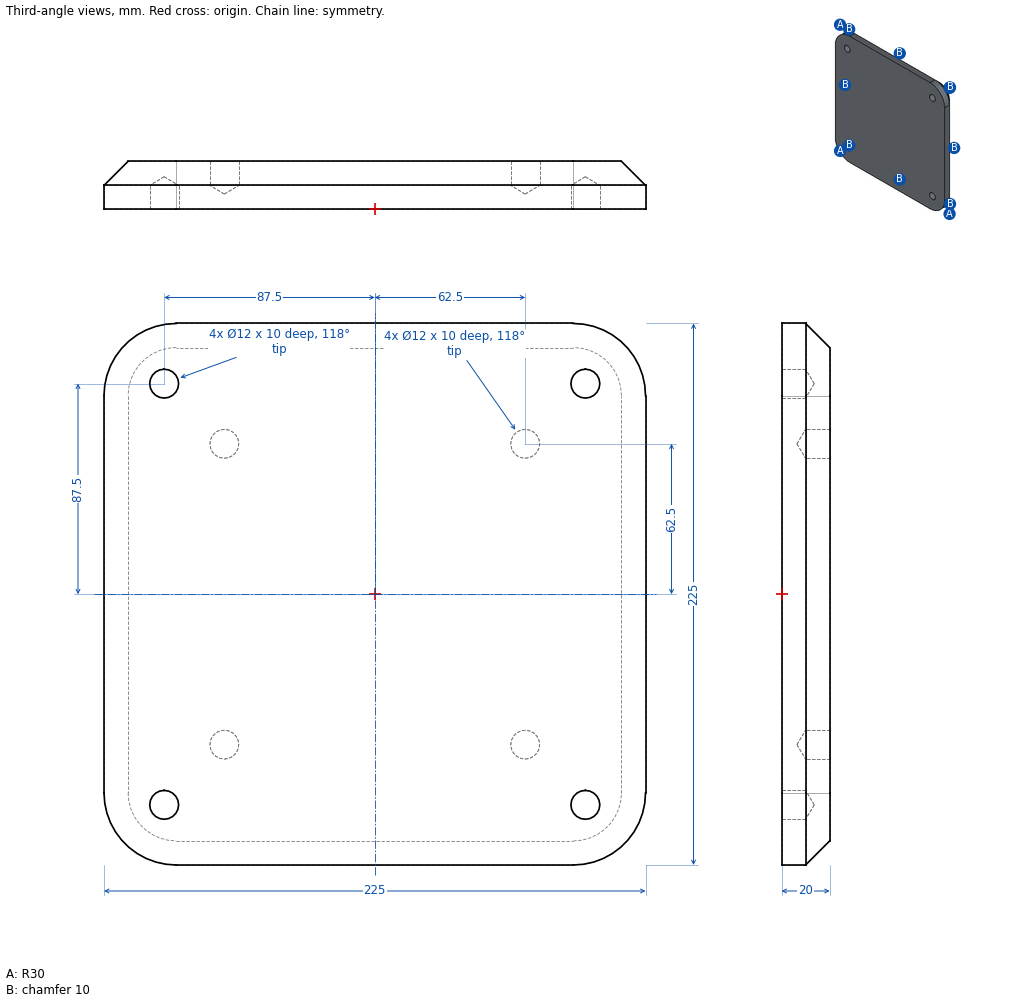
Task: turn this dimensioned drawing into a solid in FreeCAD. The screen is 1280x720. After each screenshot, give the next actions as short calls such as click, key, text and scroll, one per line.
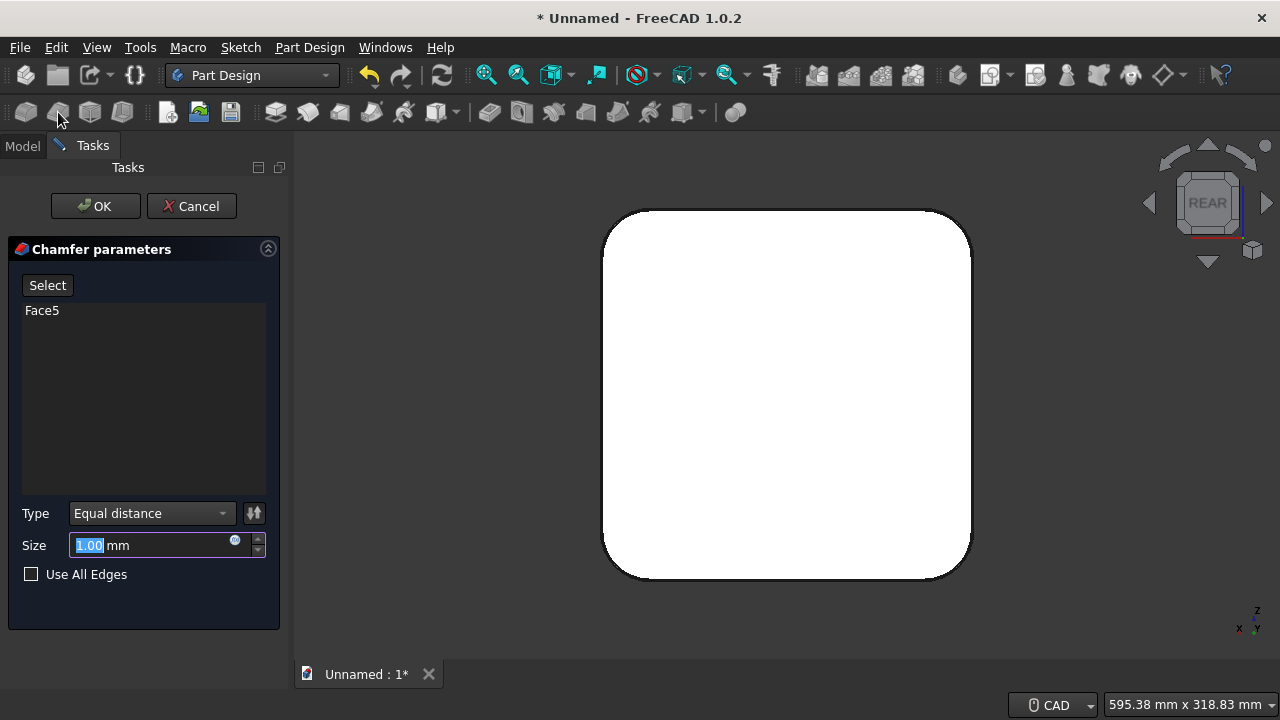
text(10)
key(Tab)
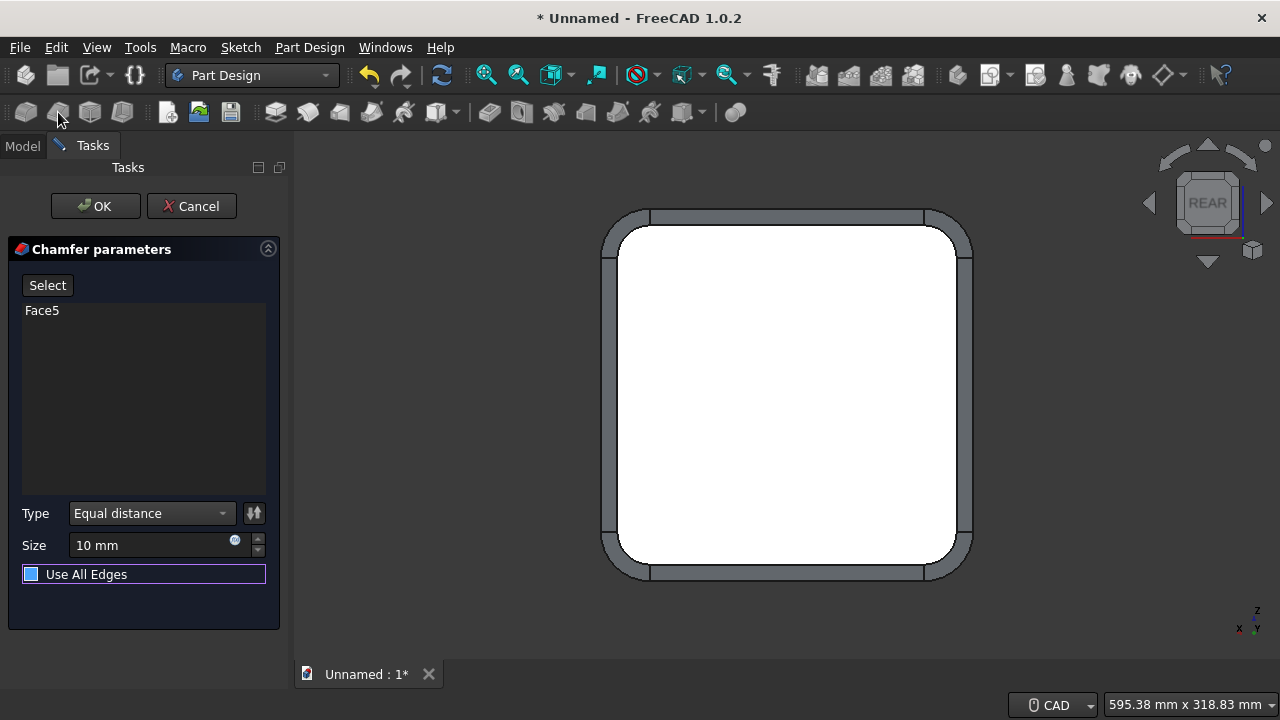
click(96, 206)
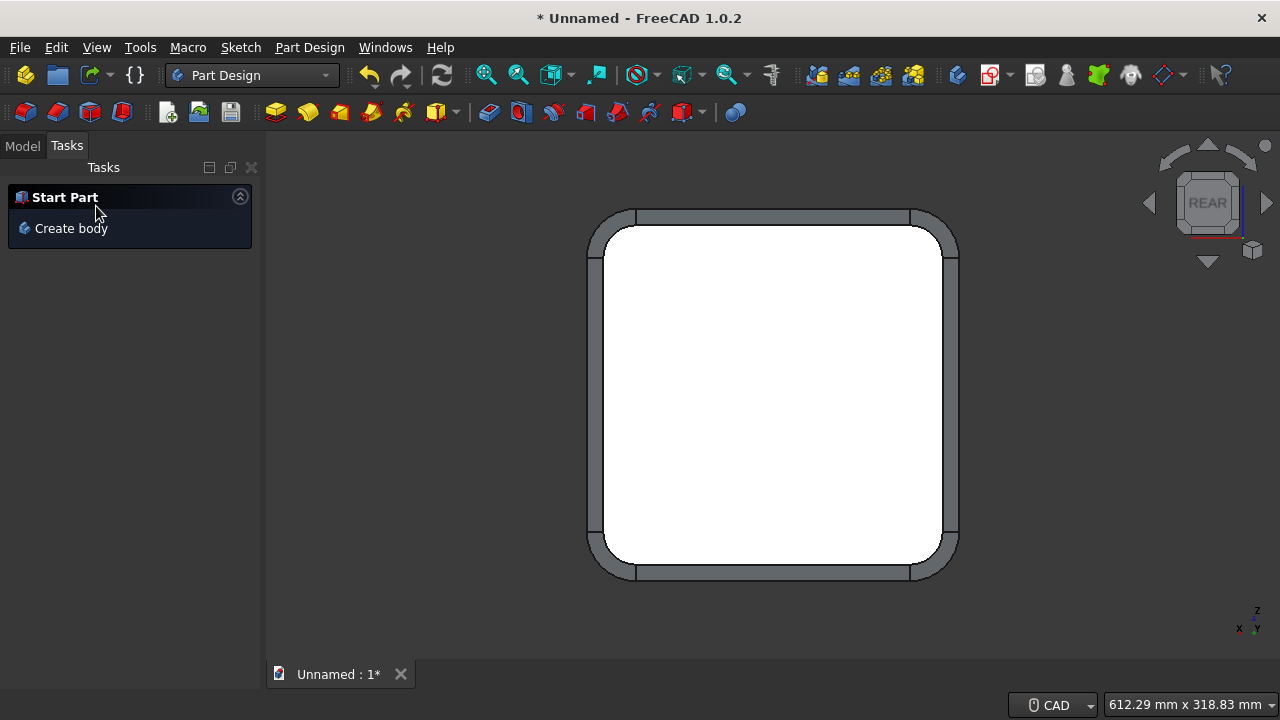
click(773, 394)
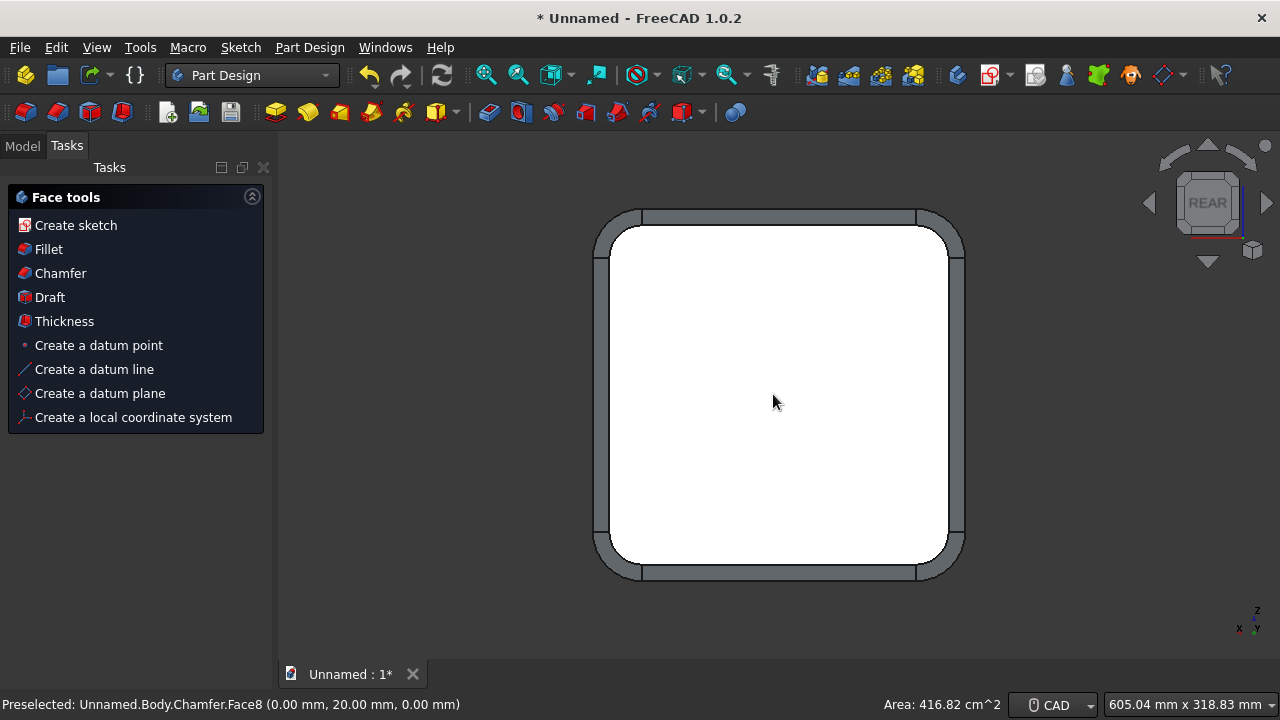
click(990, 76)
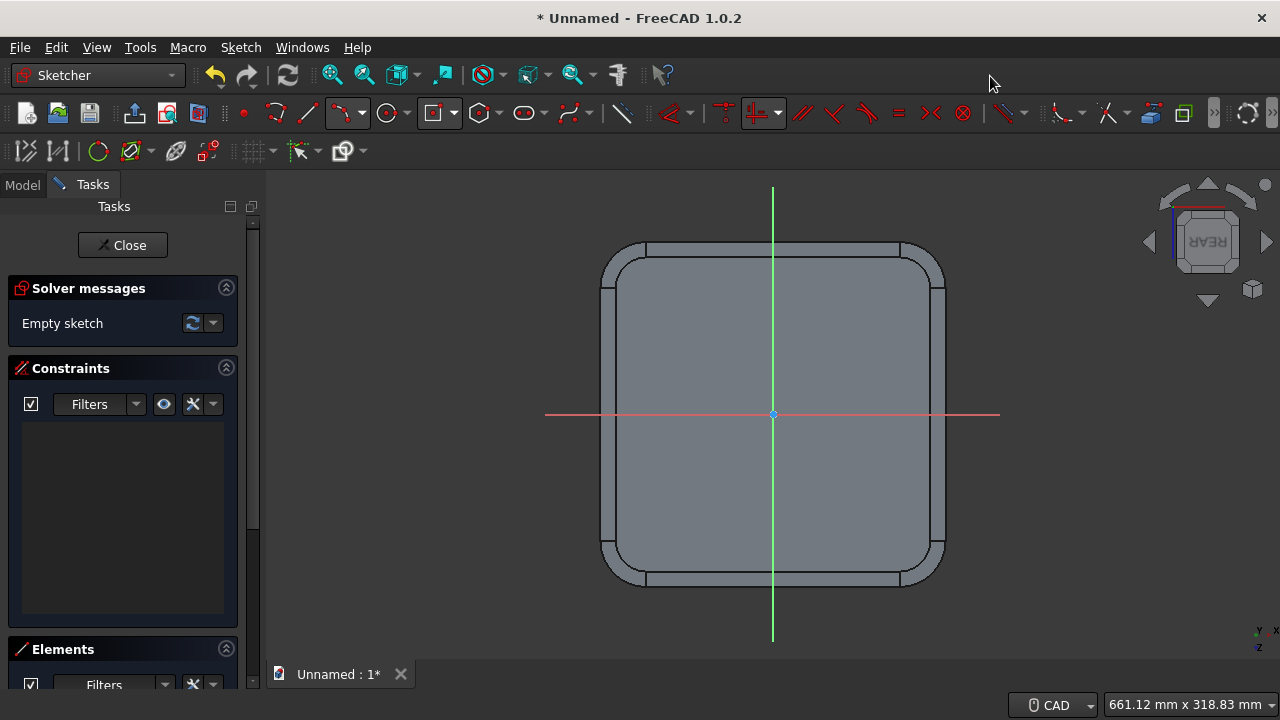
scroll(912, 415, up, 2)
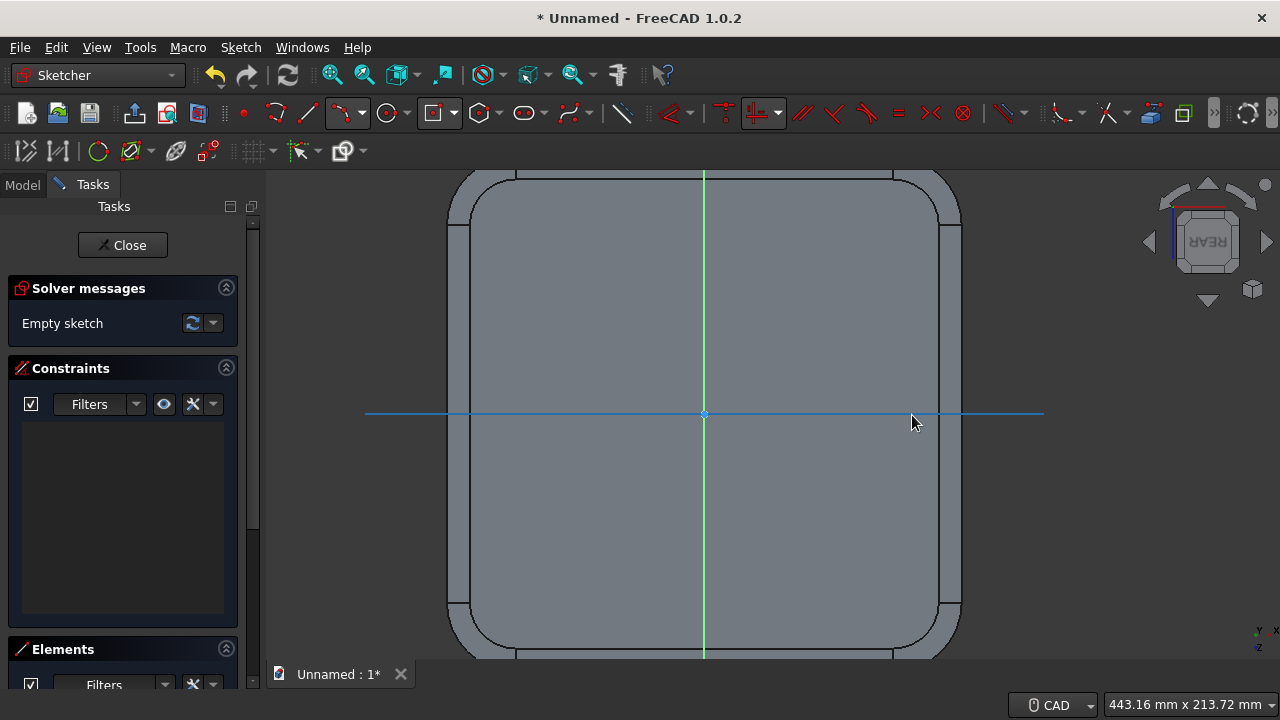
click(388, 114)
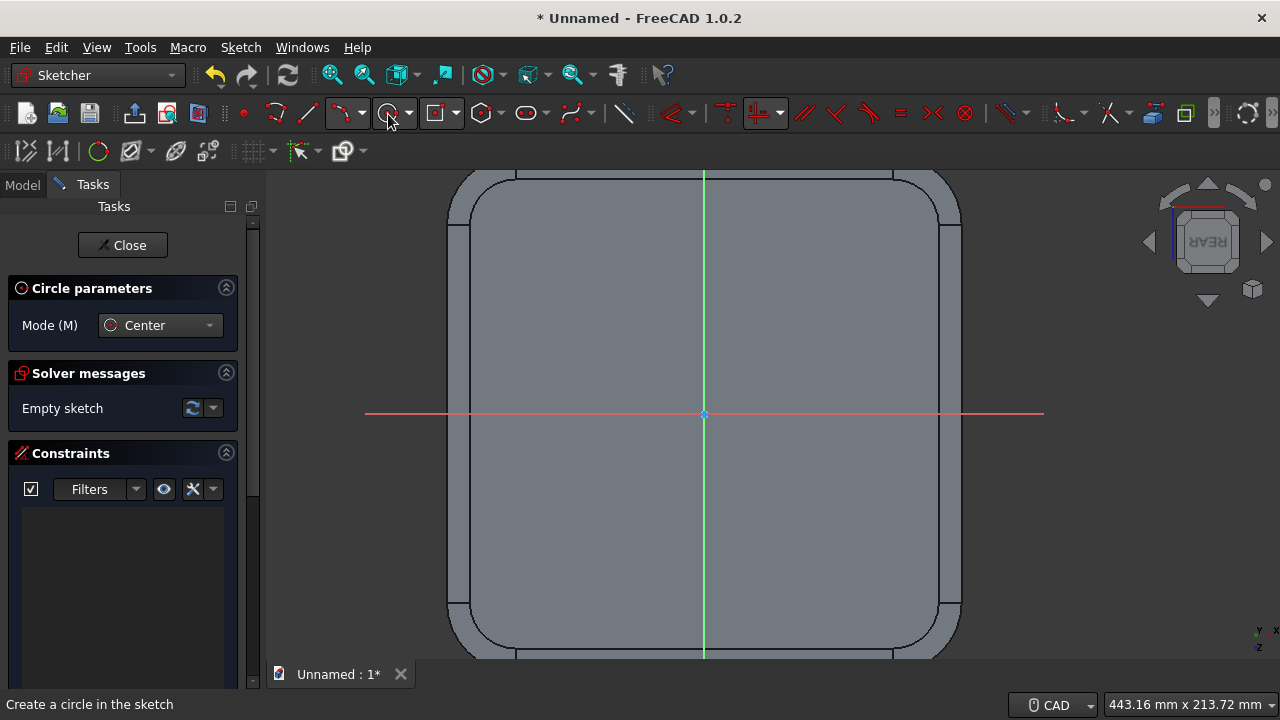
scroll(847, 557, up, 3)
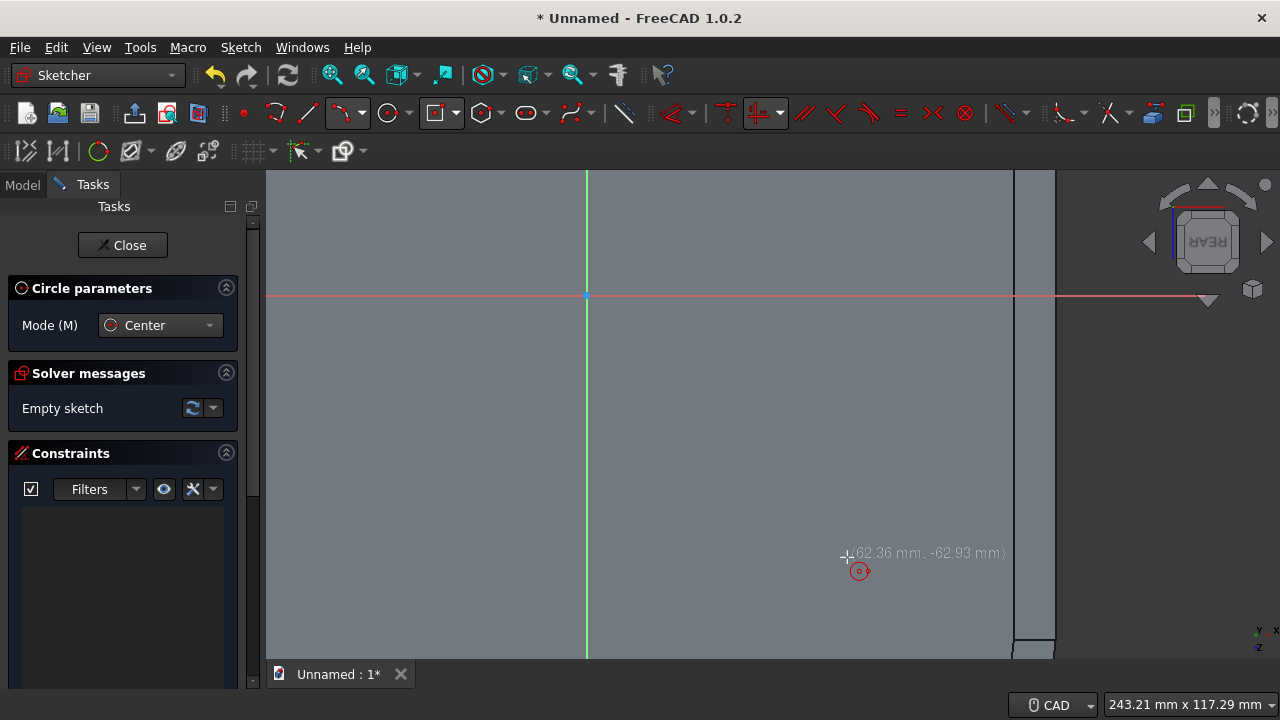
click(847, 556)
click(865, 539)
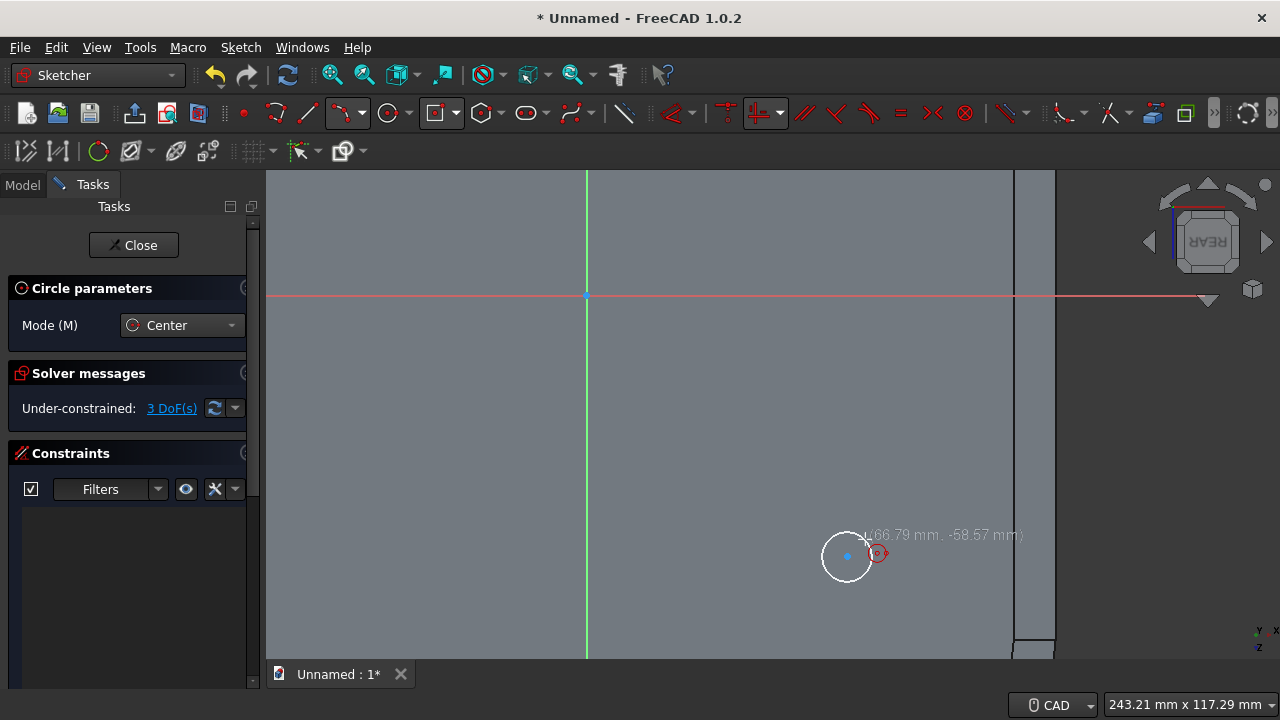
click(326, 556)
click(344, 539)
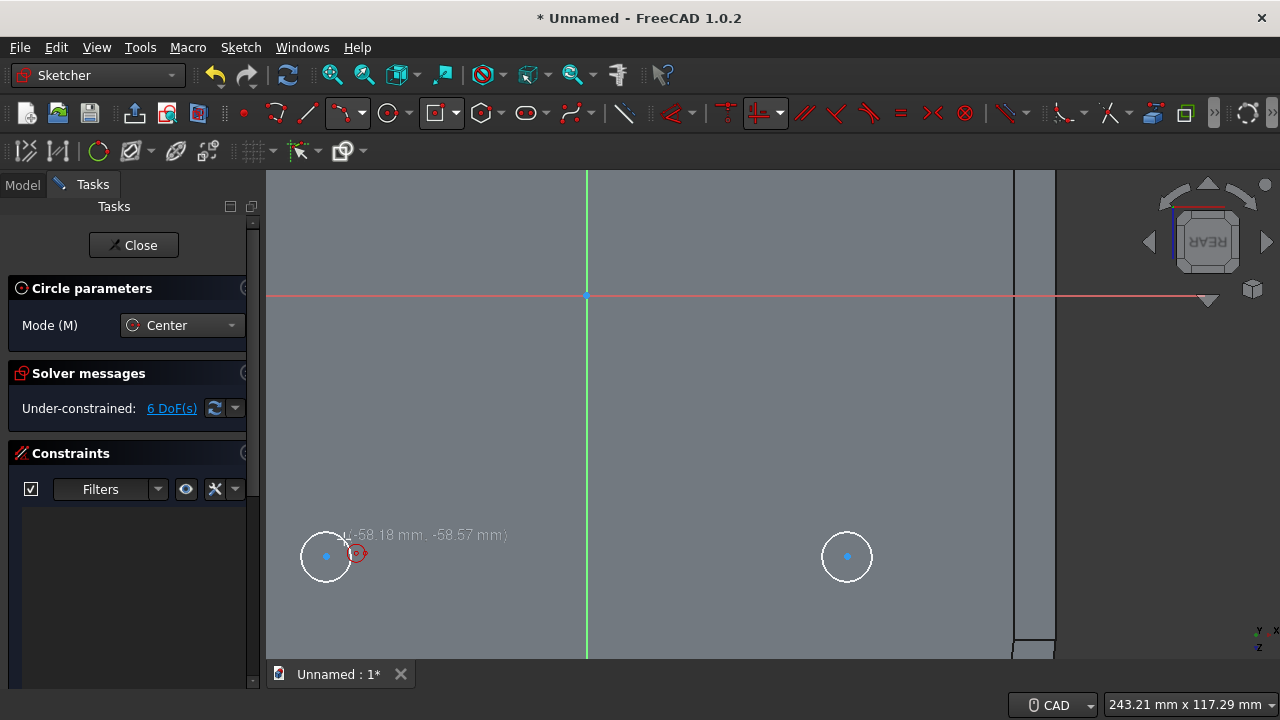
scroll(848, 559, down, 3)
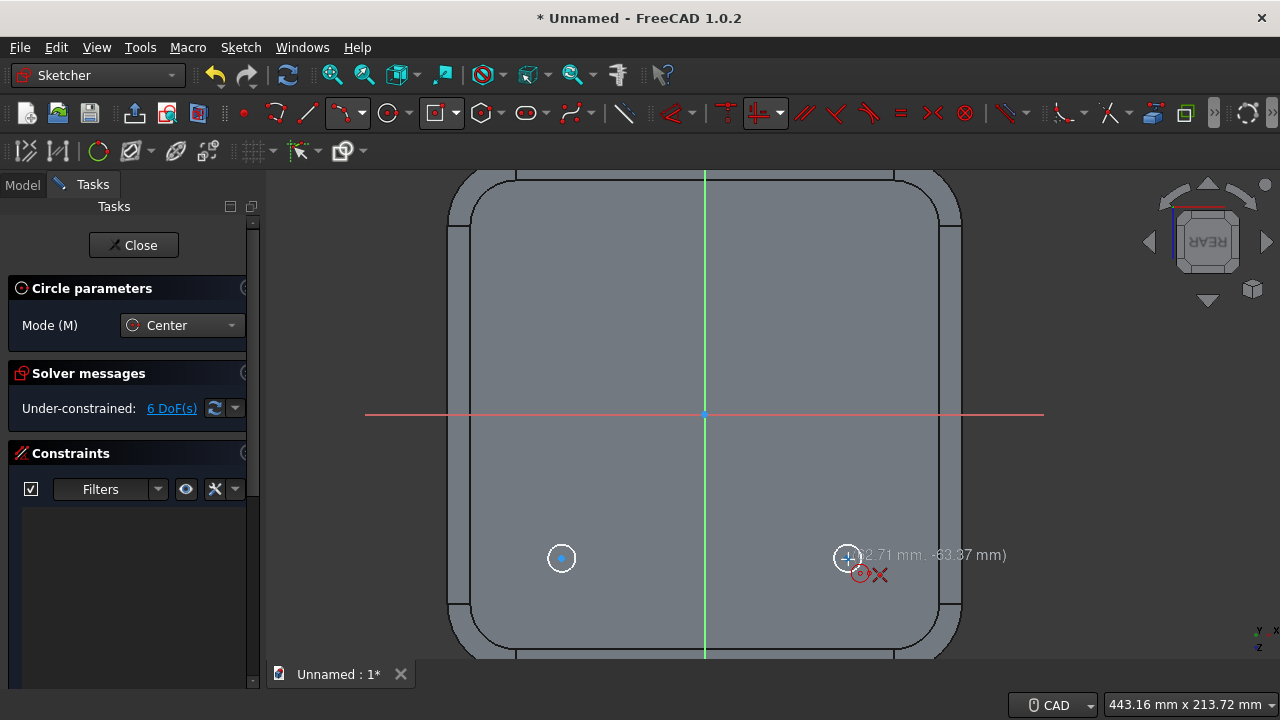
scroll(562, 272, up, 3)